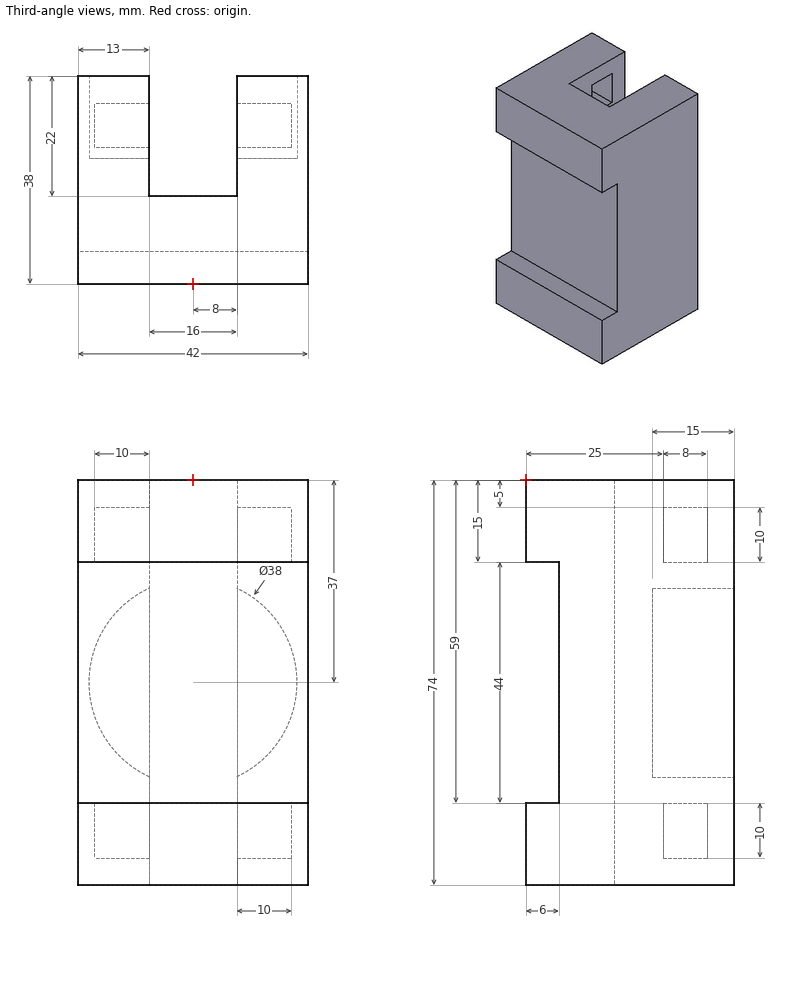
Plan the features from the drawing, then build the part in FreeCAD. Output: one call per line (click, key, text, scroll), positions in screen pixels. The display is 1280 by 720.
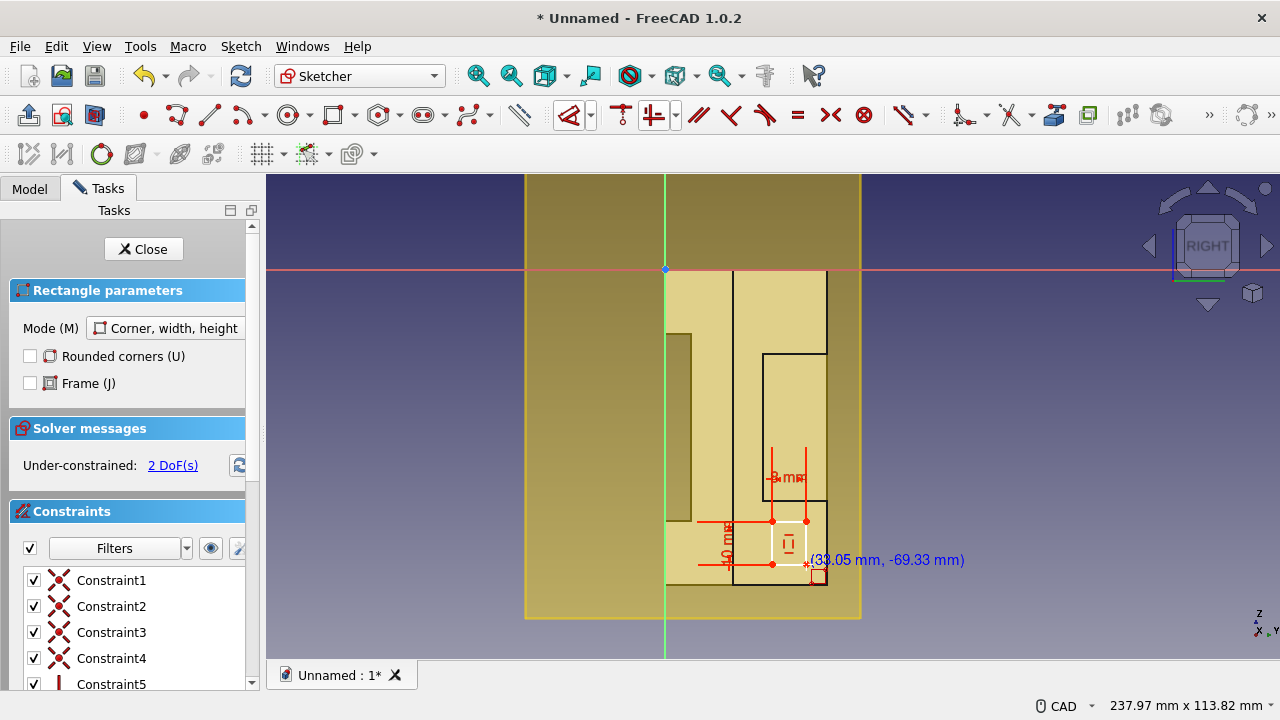
click(772, 291)
move(806, 334)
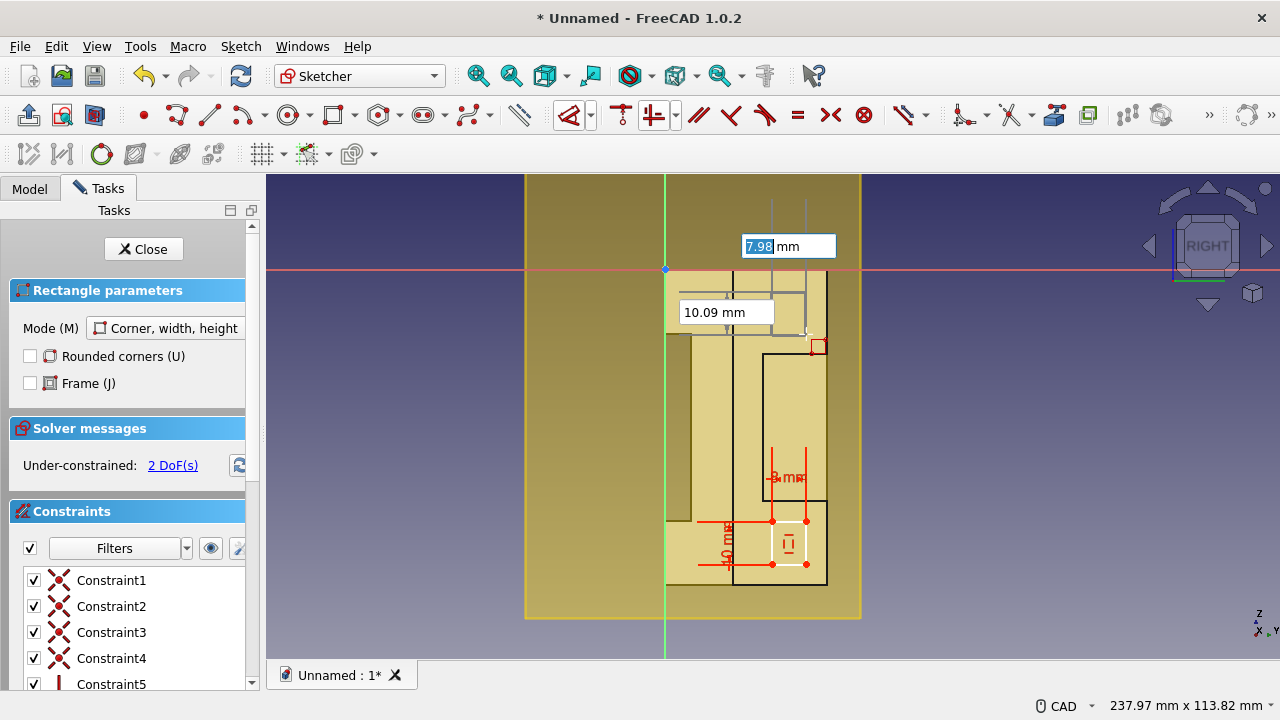
text(8)
key(Tab)
text(10)
key(Return)
key(Escape)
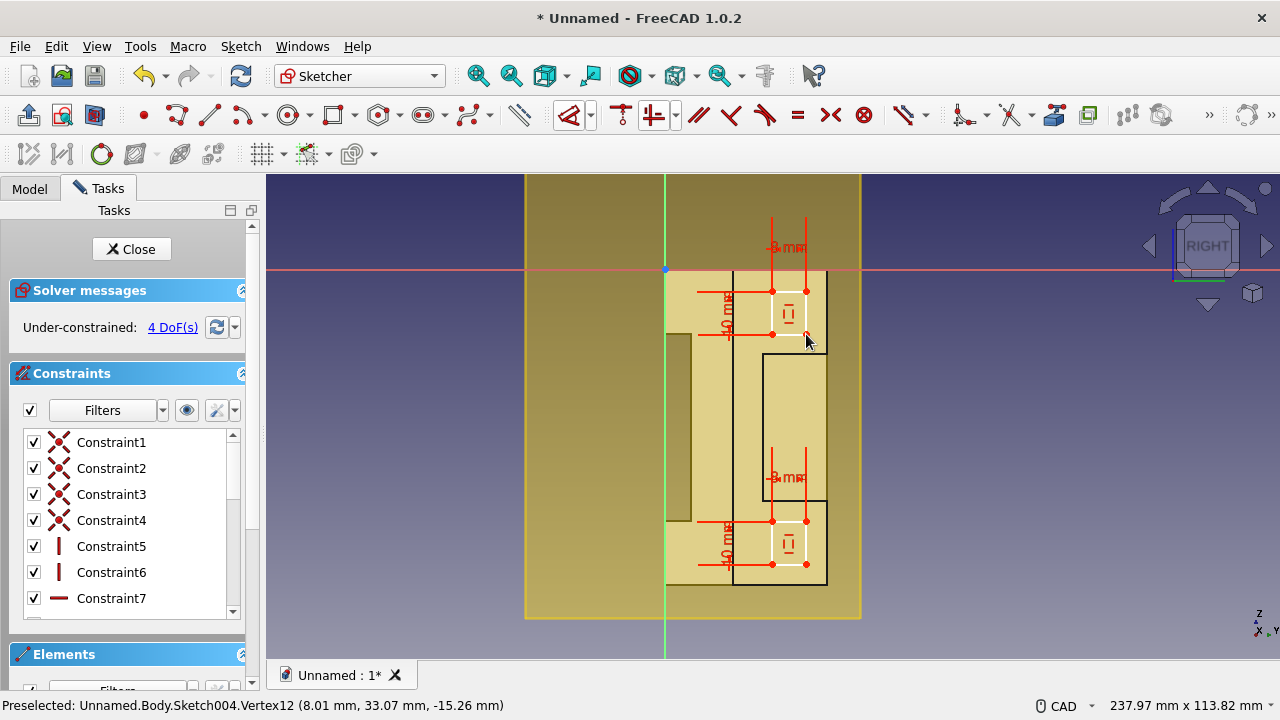
scroll(772, 292, up, 4)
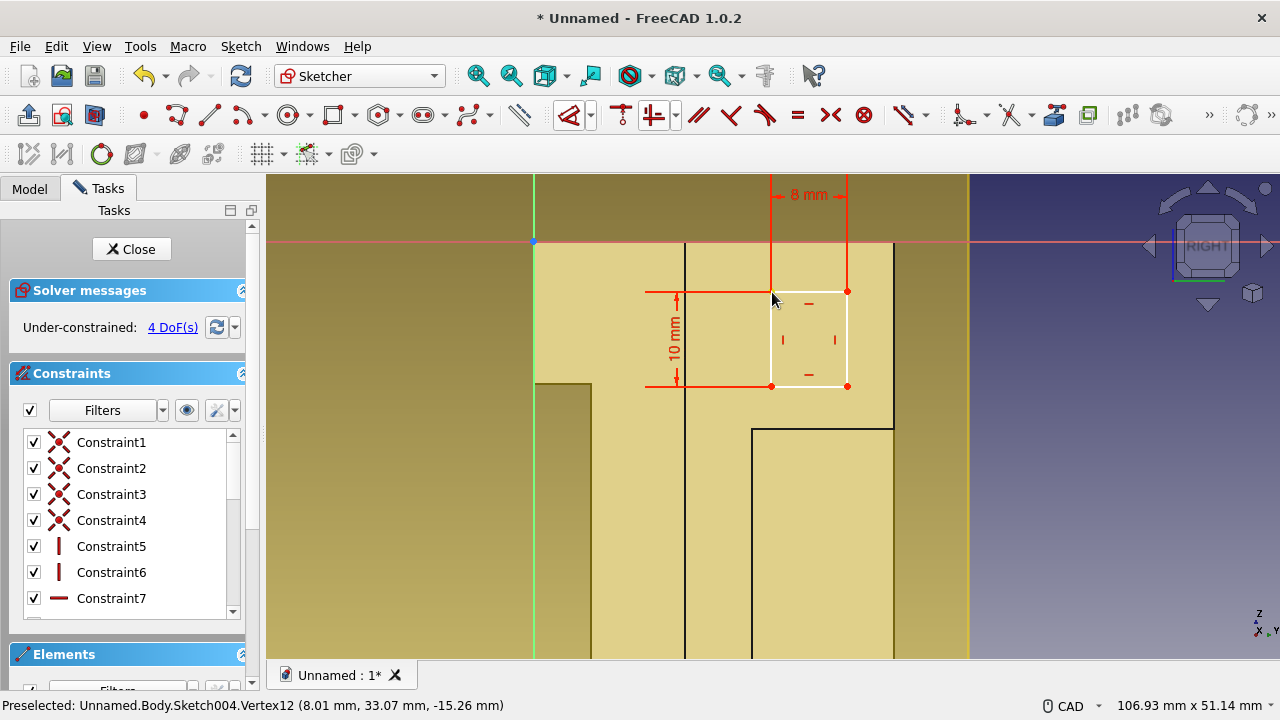
click(771, 292)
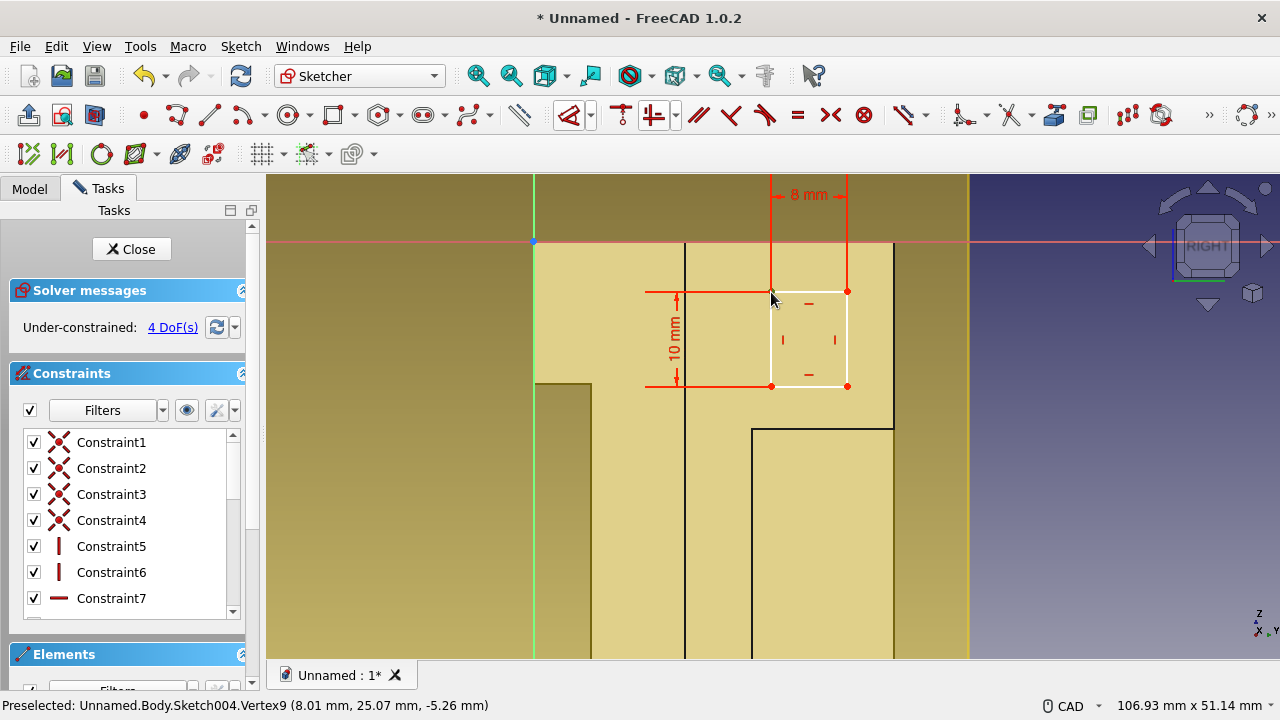
key(i)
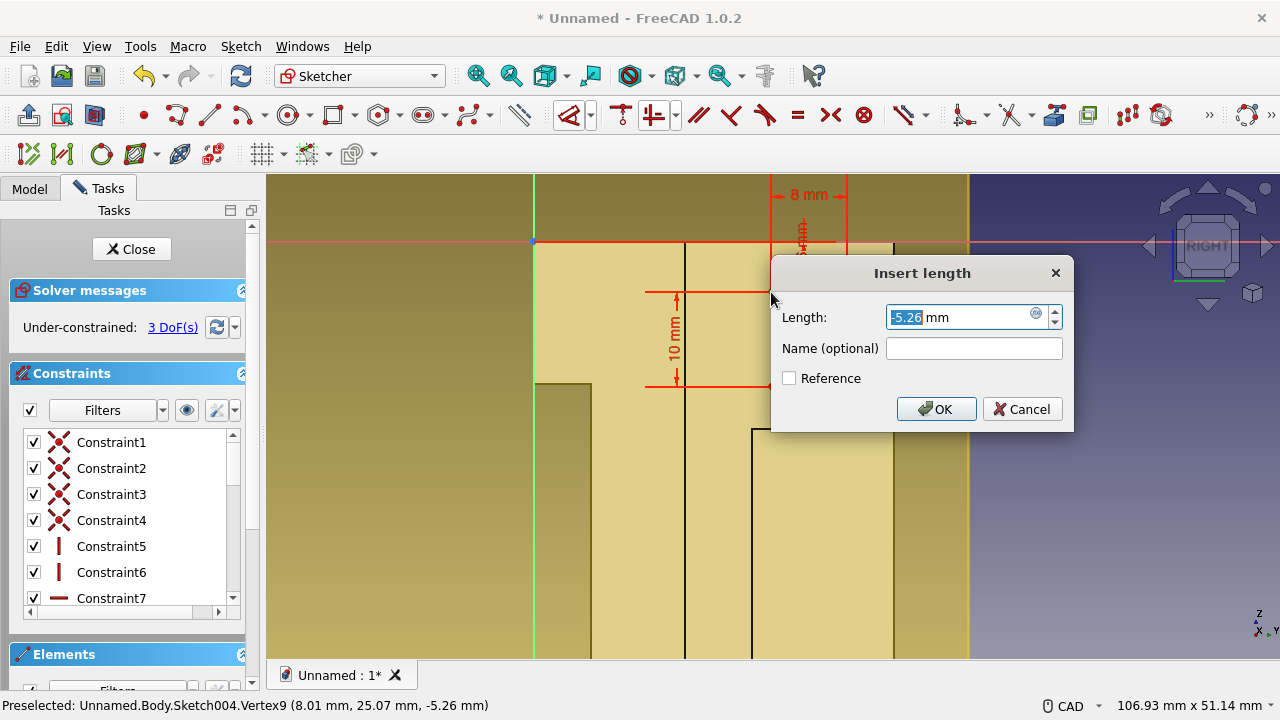
text(-5)
key(Return)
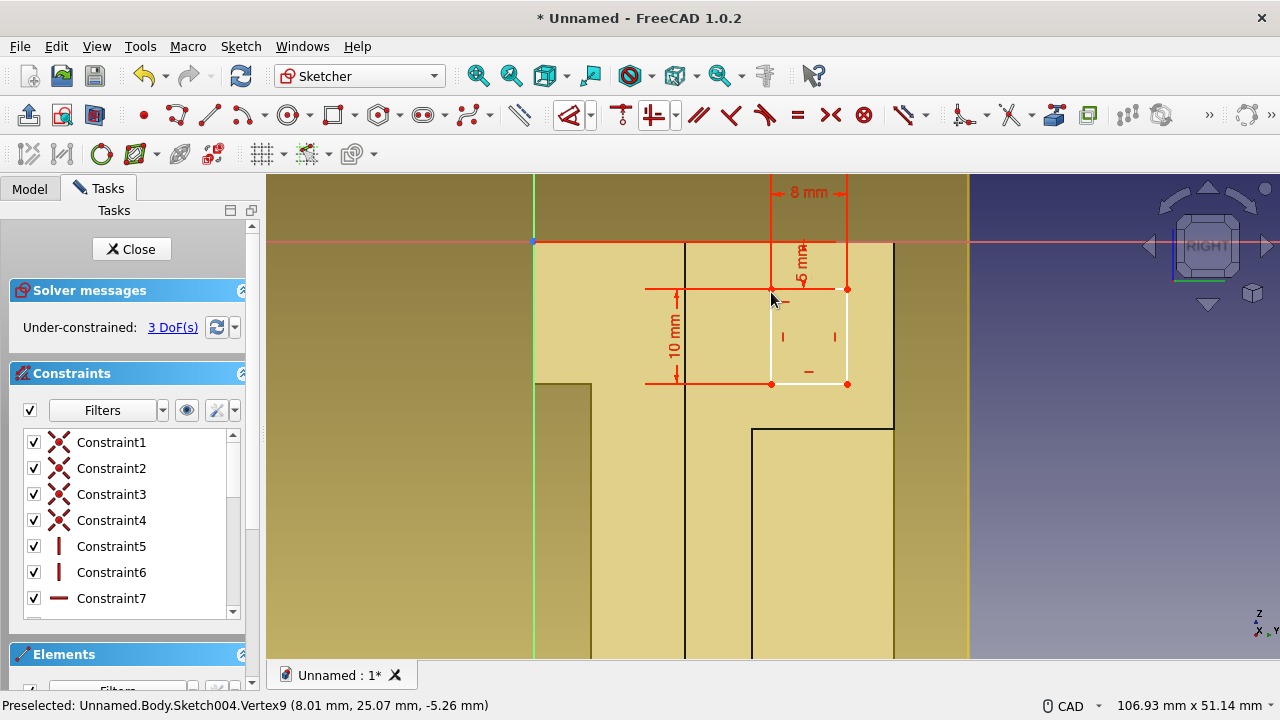
scroll(716, 292, down, 4)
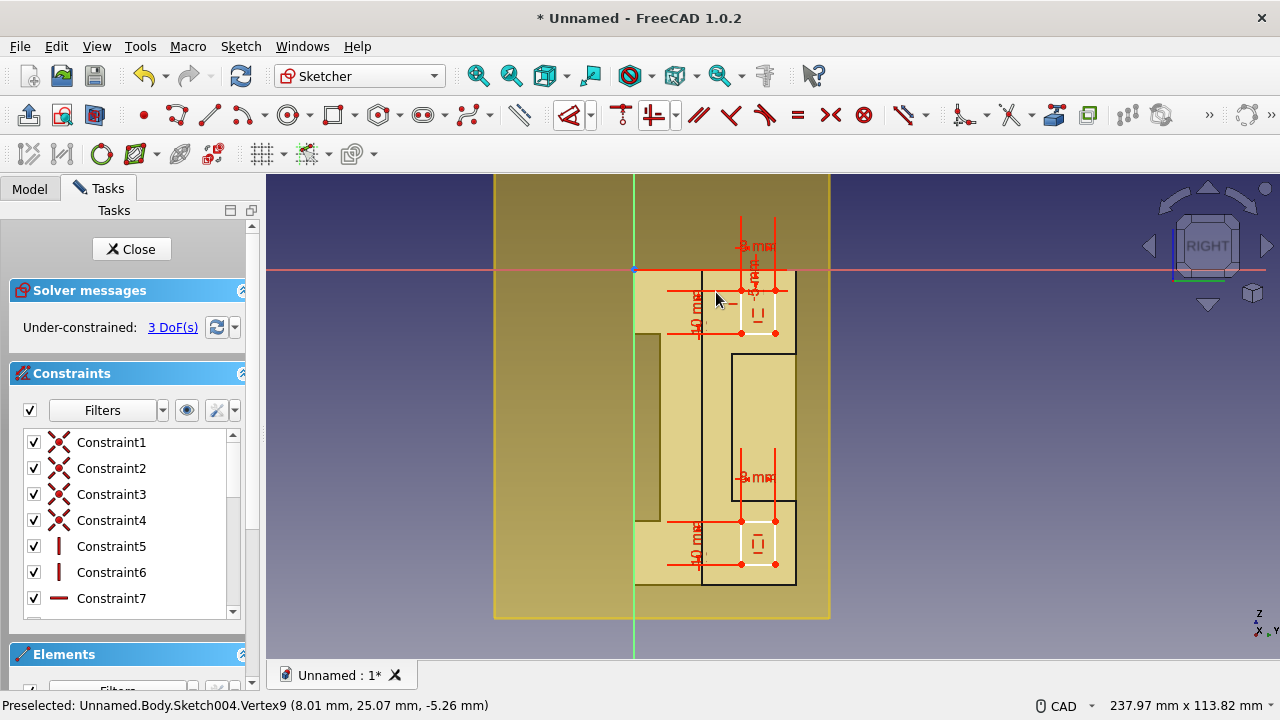
click(741, 522)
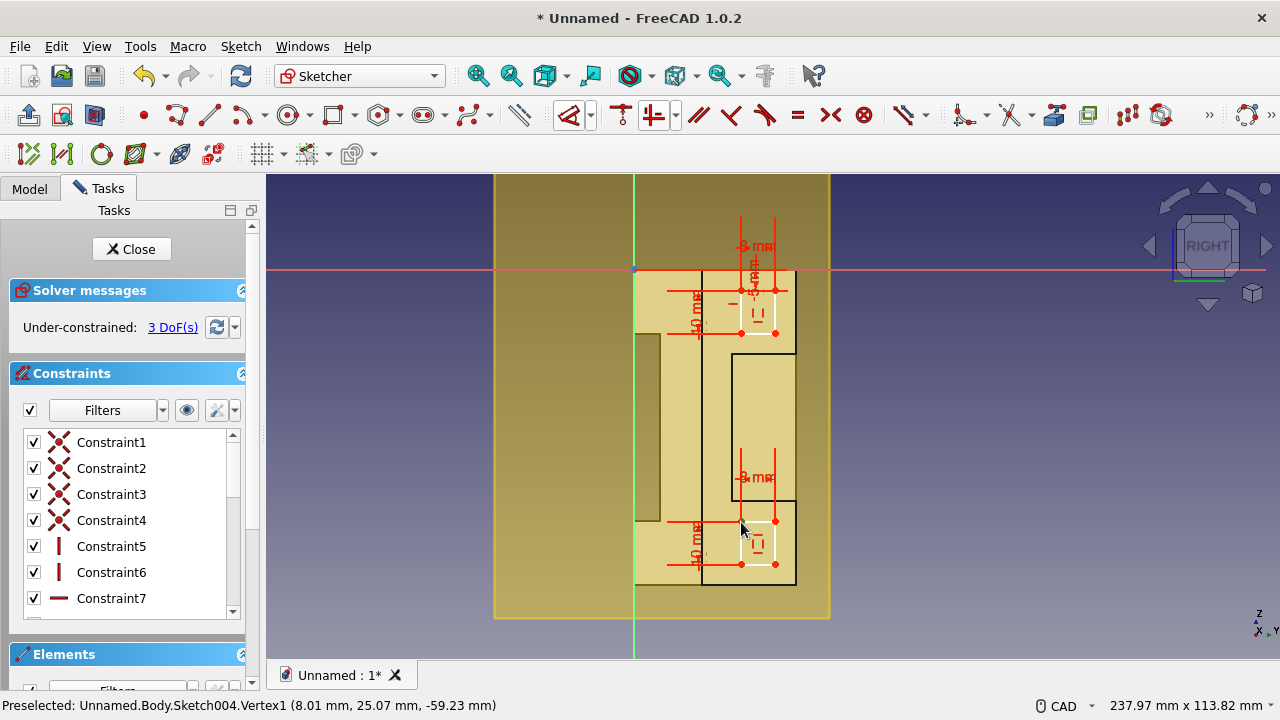
key(l)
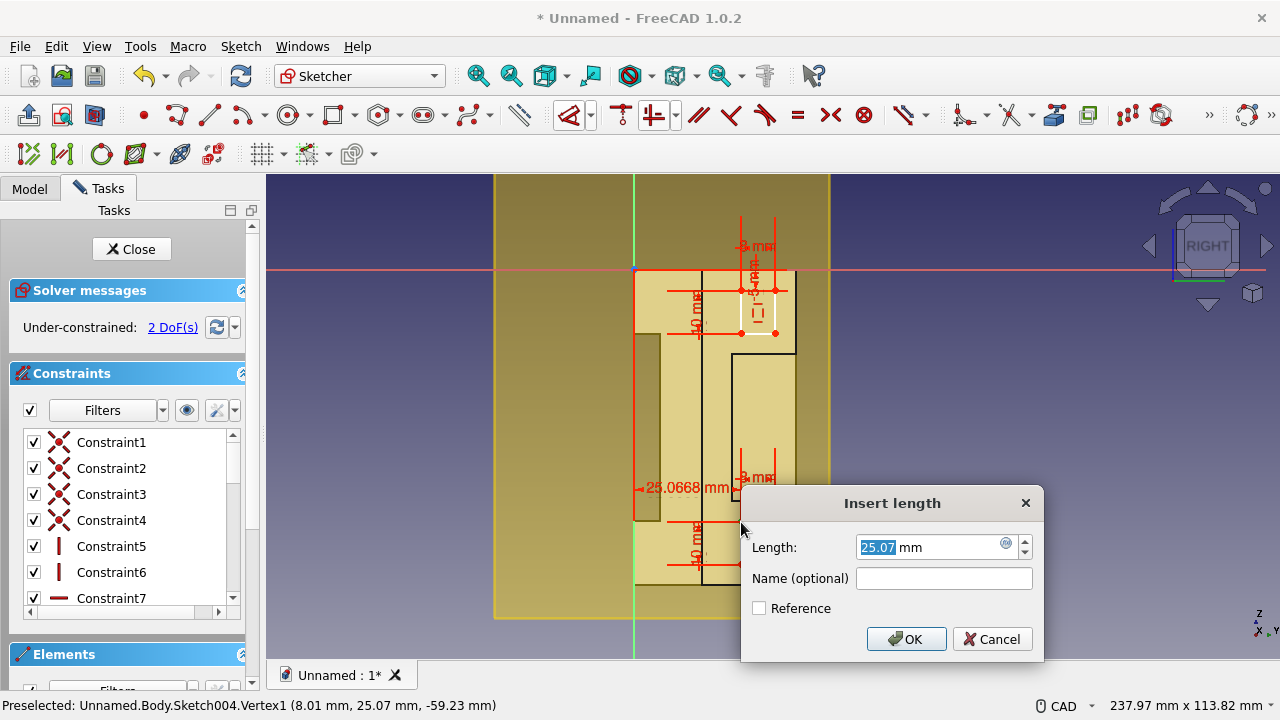
text(25)
key(Return)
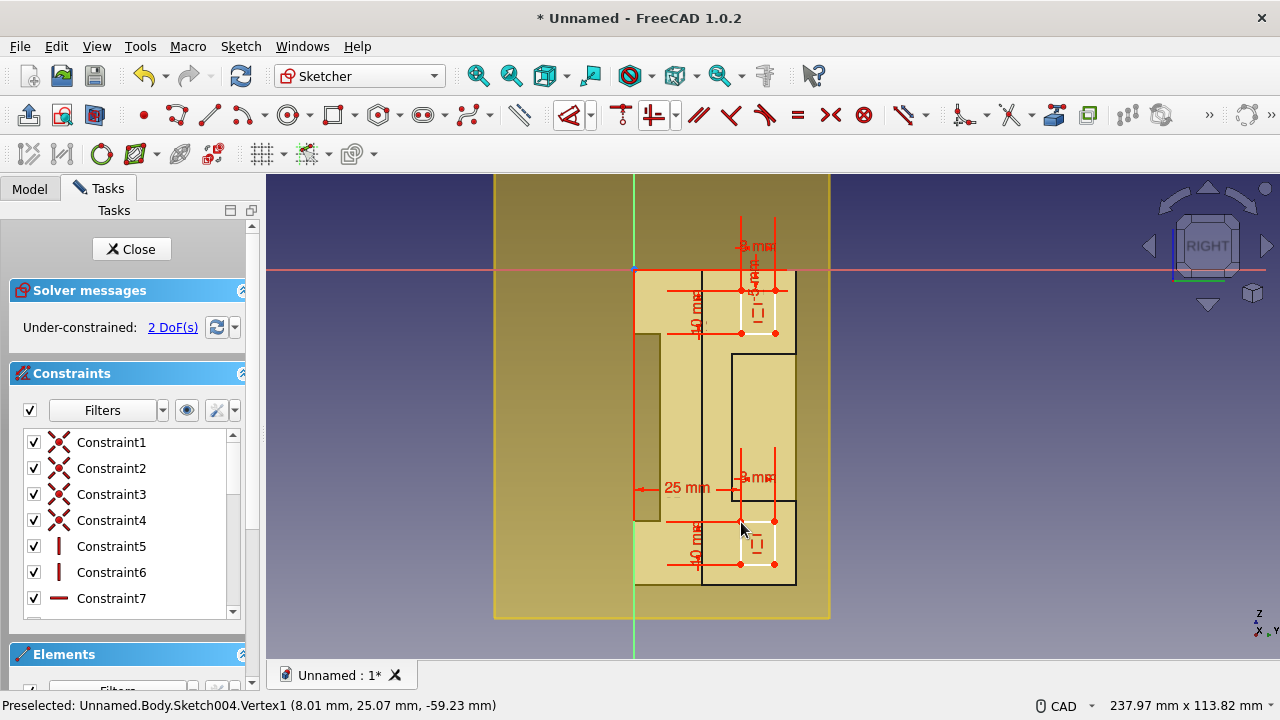
click(741, 522)